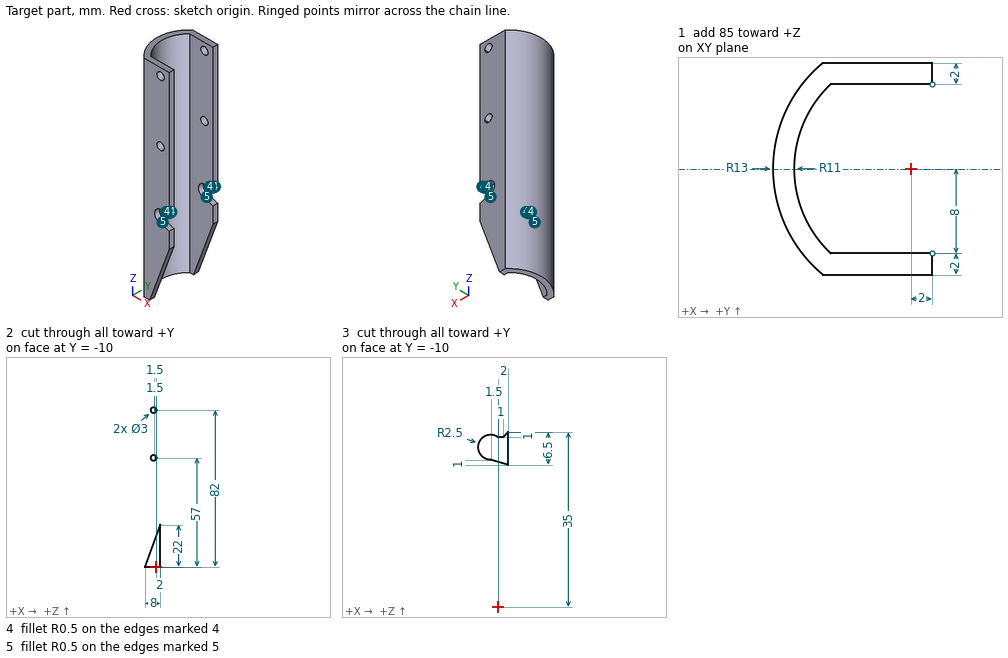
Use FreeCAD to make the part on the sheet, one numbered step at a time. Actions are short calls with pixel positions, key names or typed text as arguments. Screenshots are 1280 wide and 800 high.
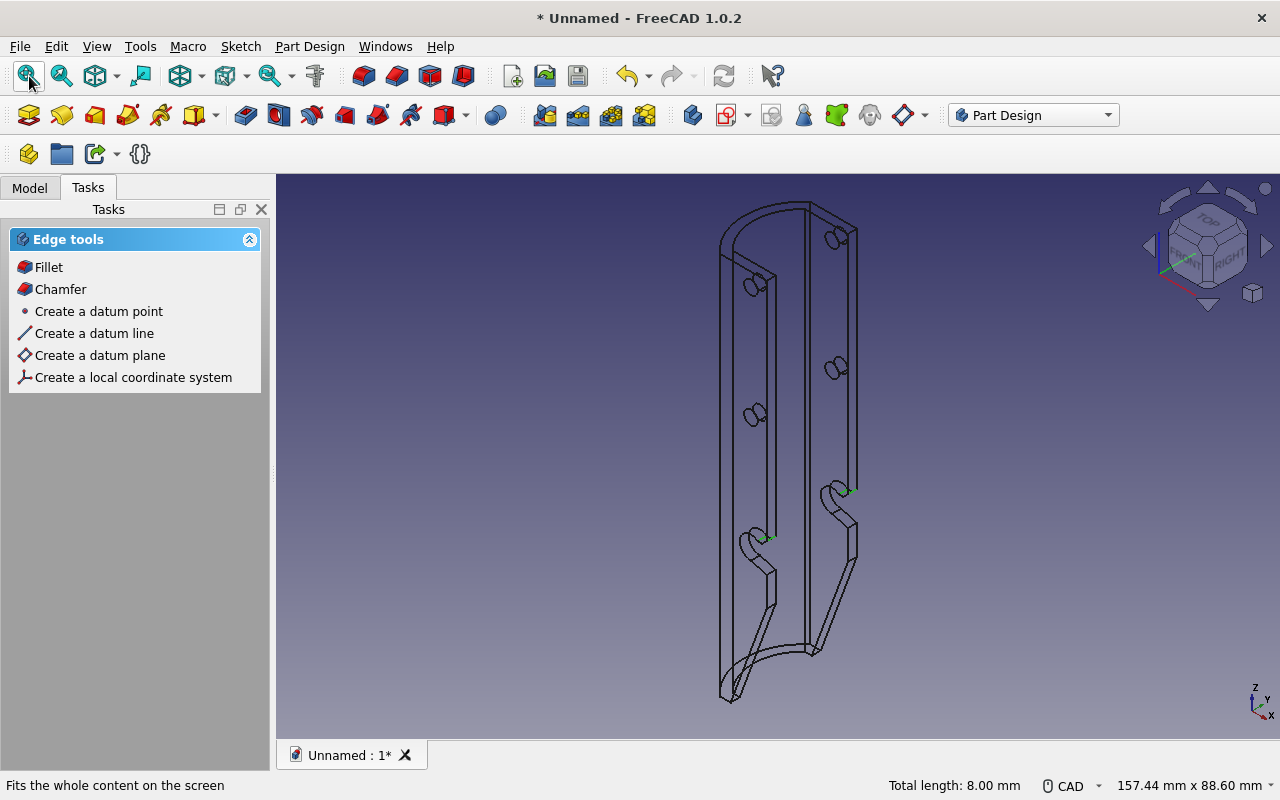
key(2)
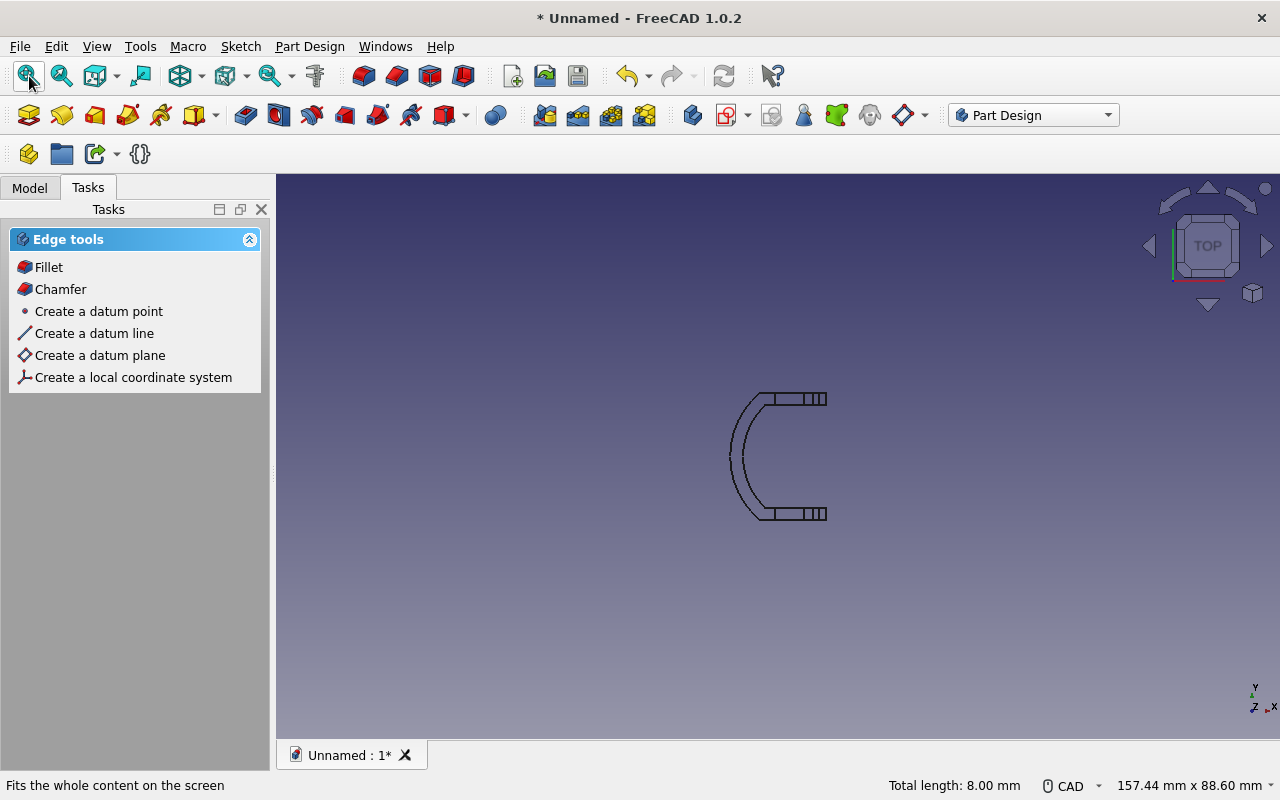
click(29, 76)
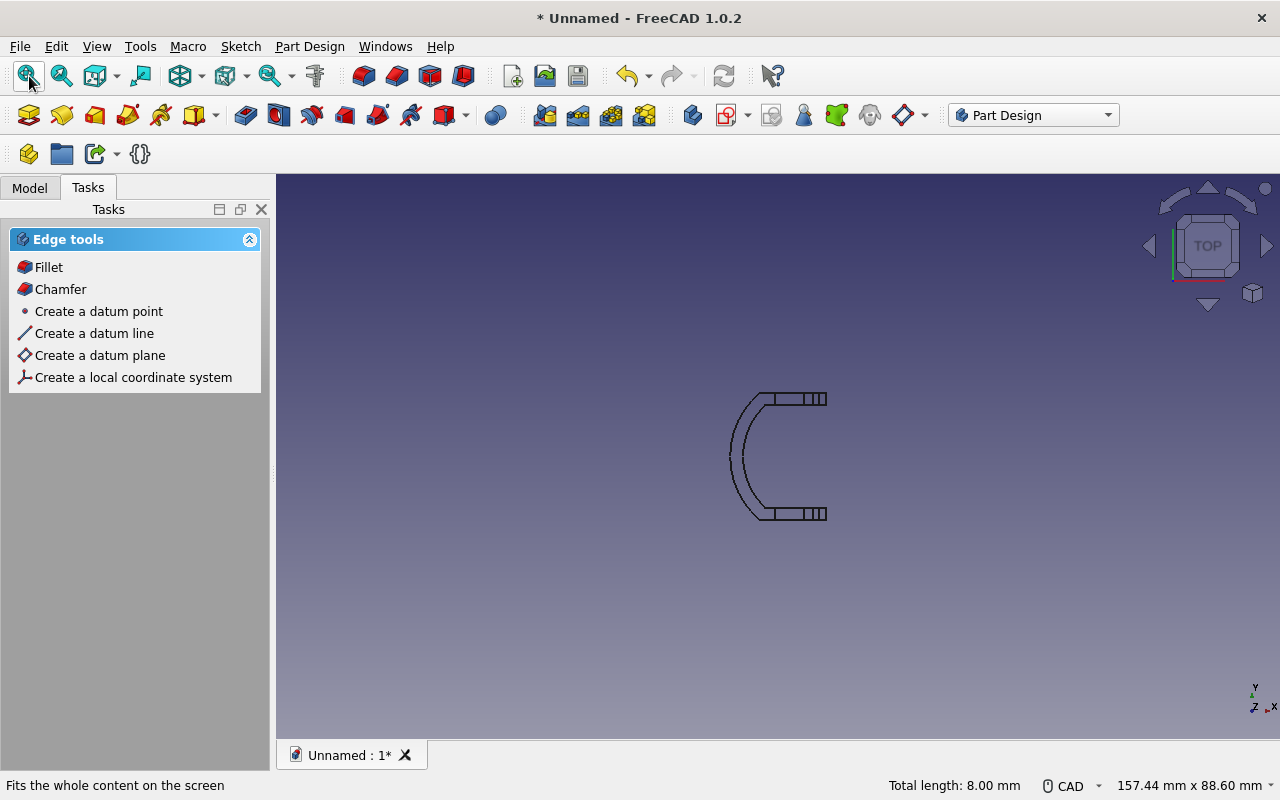
scroll(819, 513, up, 6)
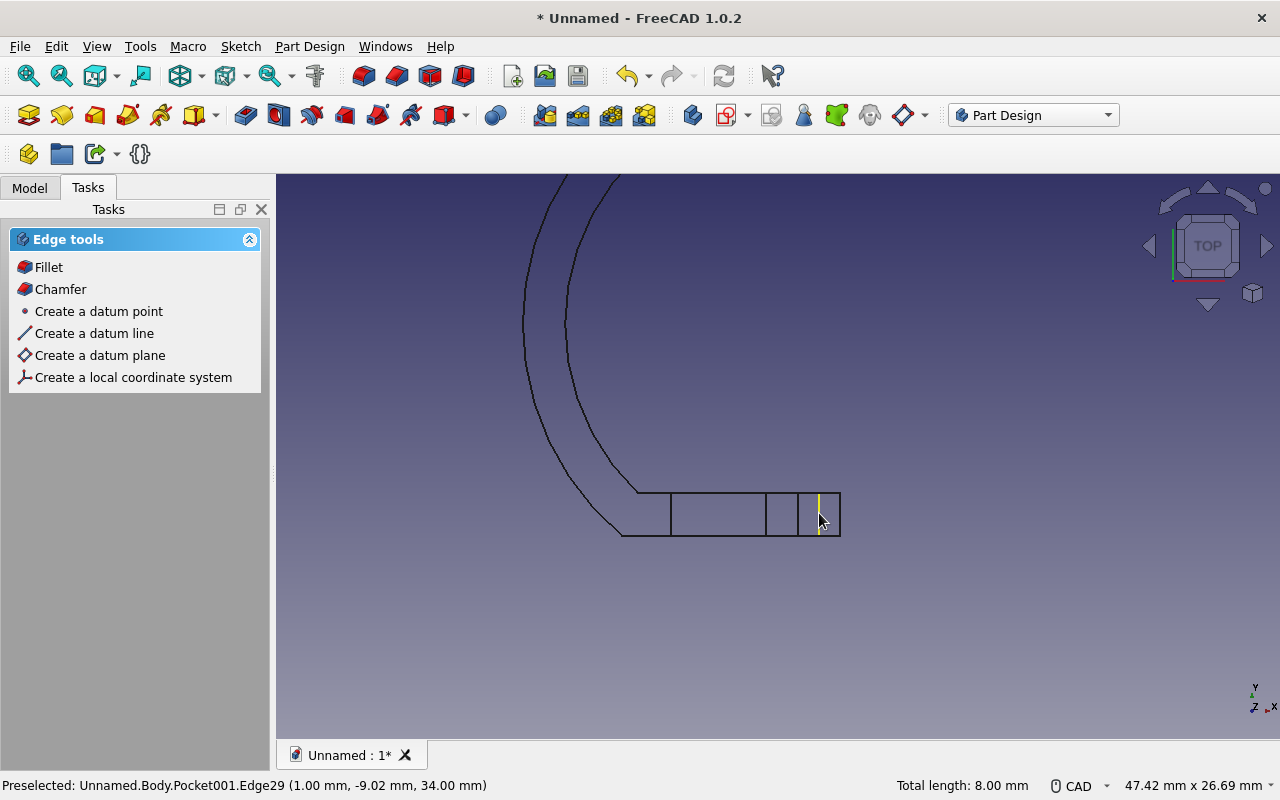
click(819, 514, ctrl)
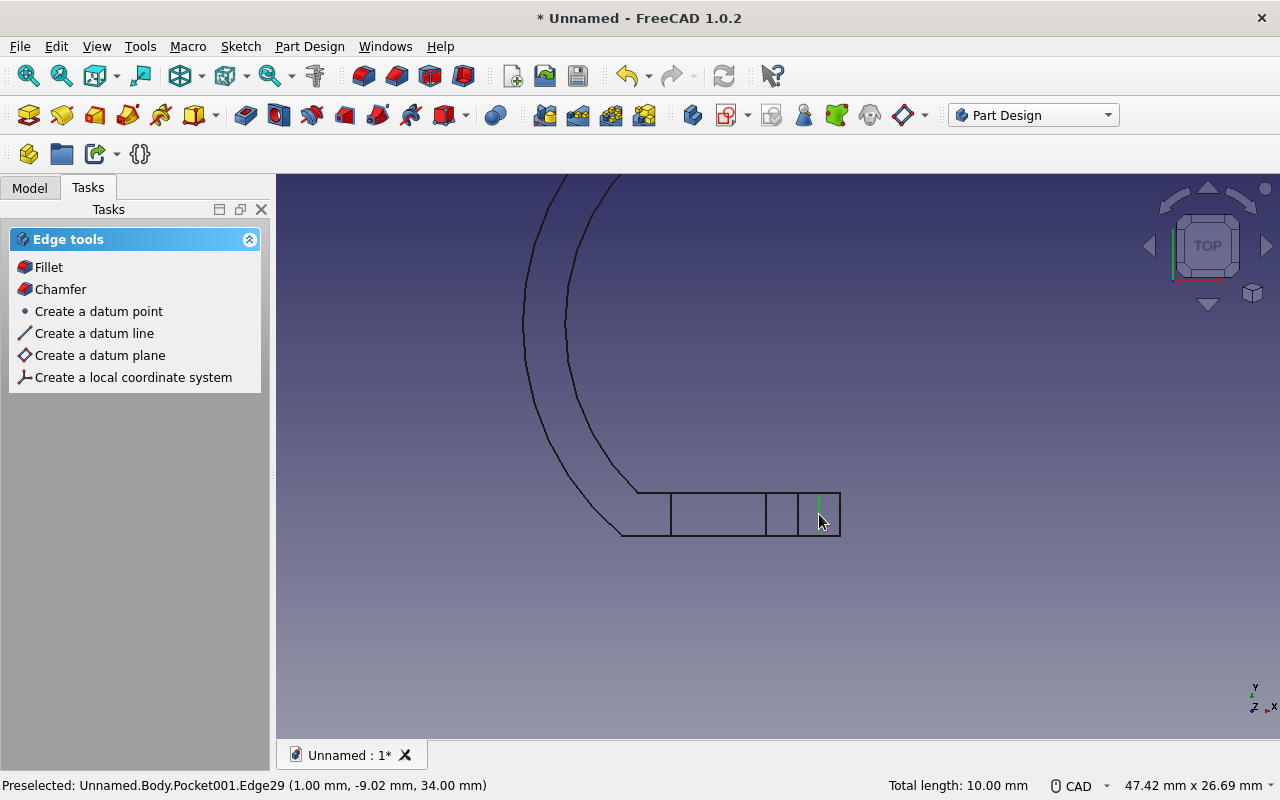
key(v)
key(f)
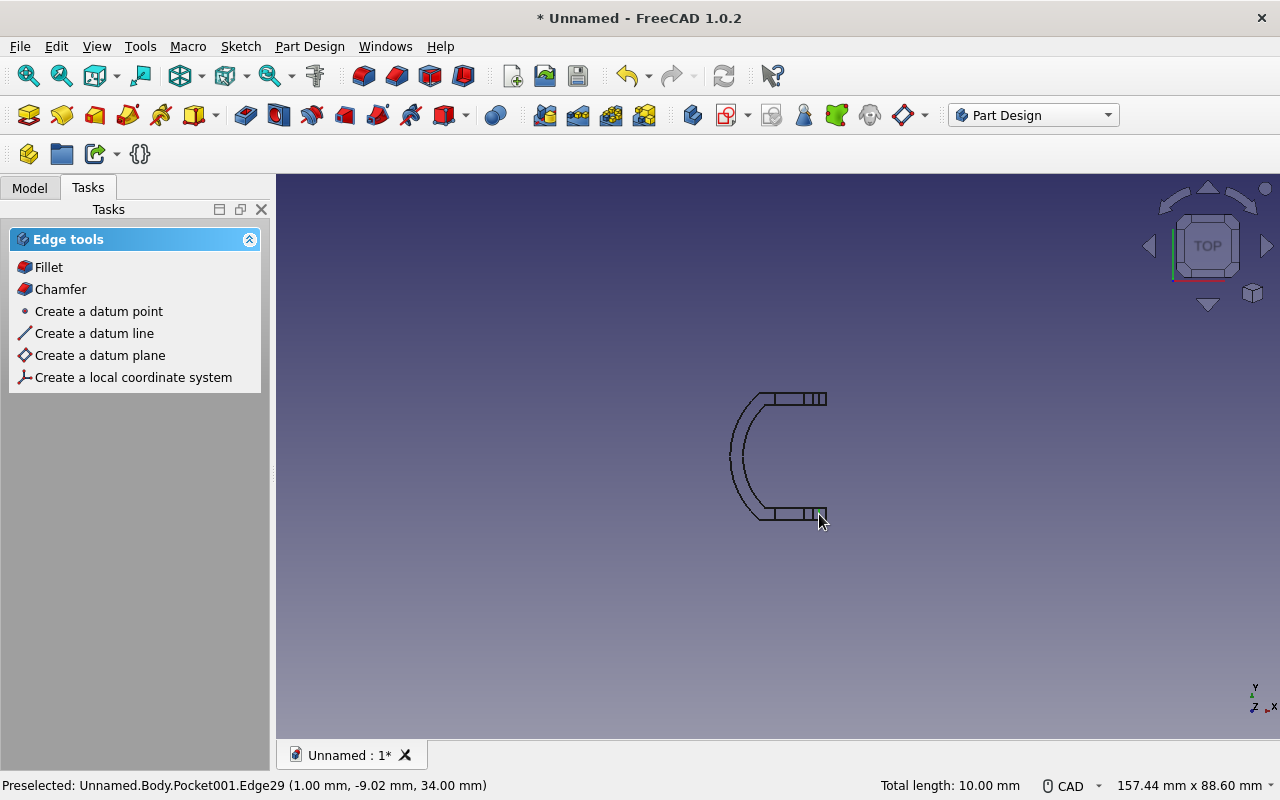
key(1)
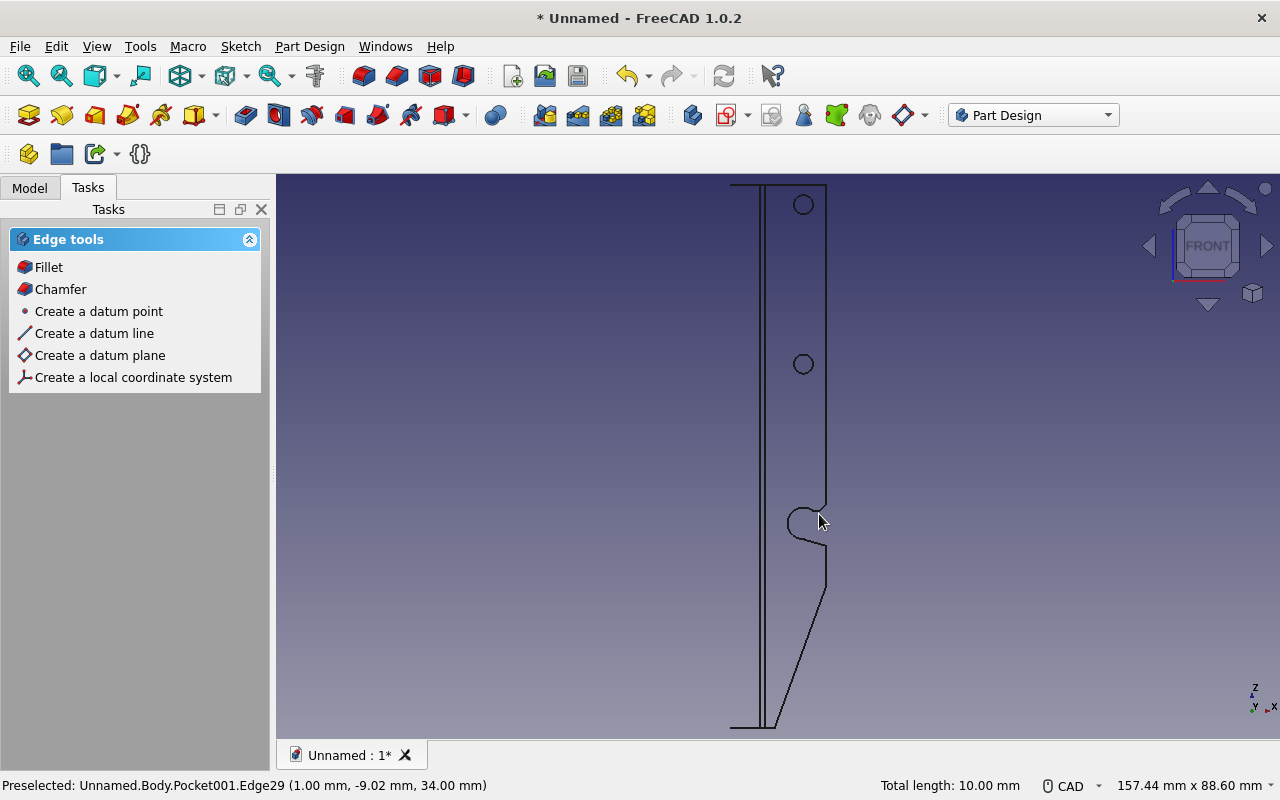
scroll(819, 510, up, 6)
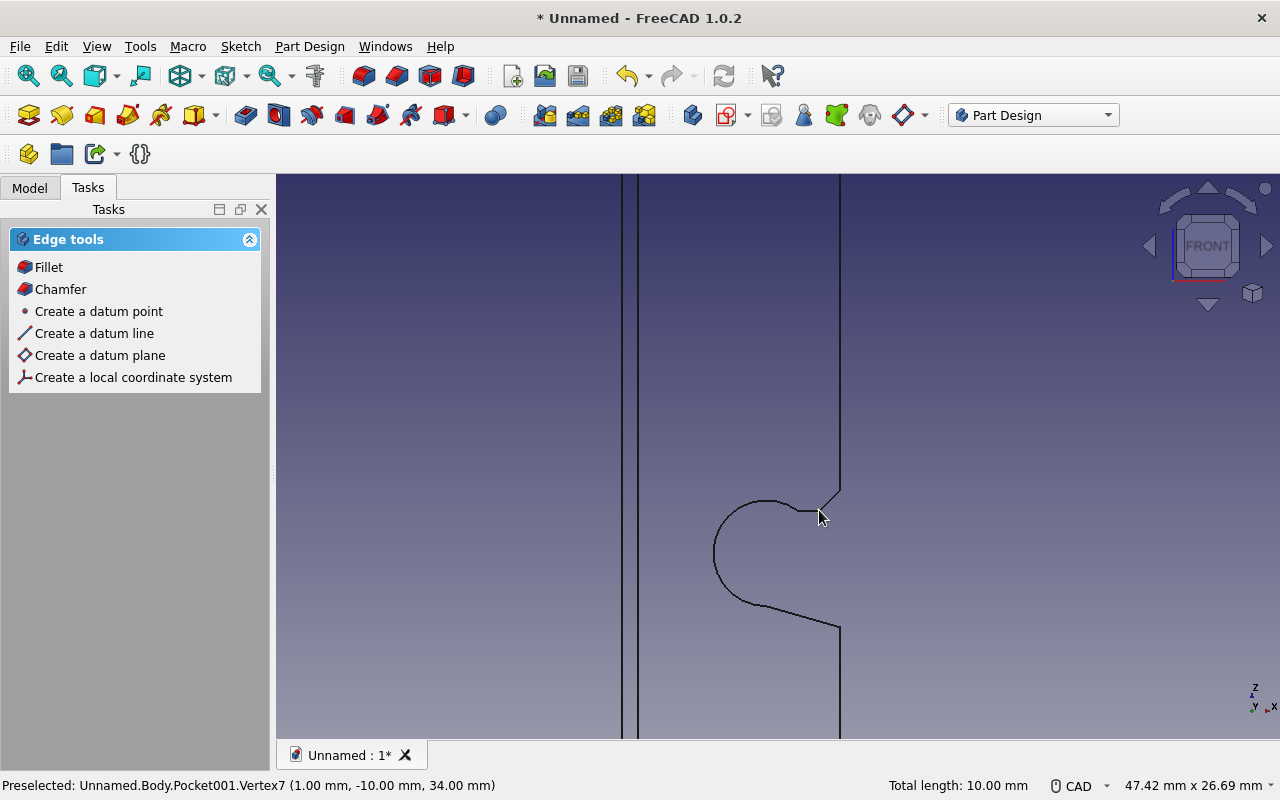
click(29, 76)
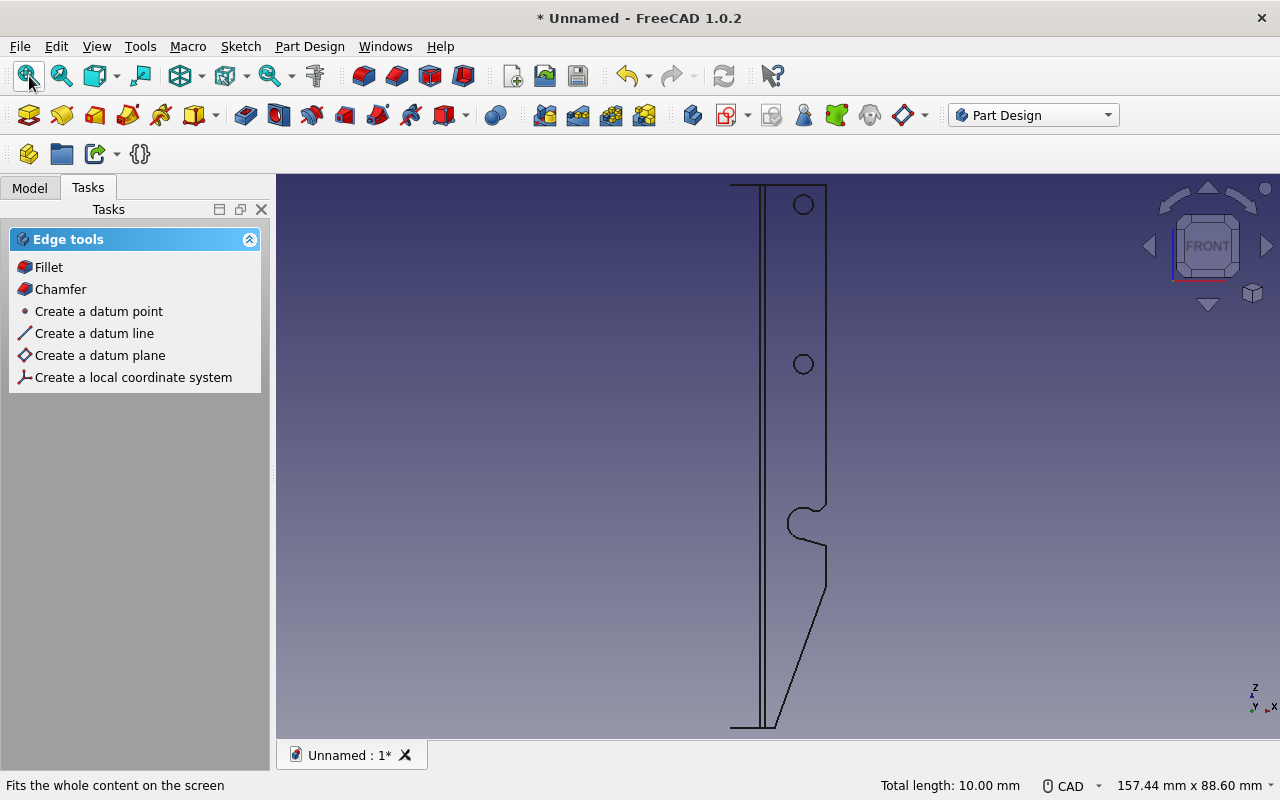
key(3)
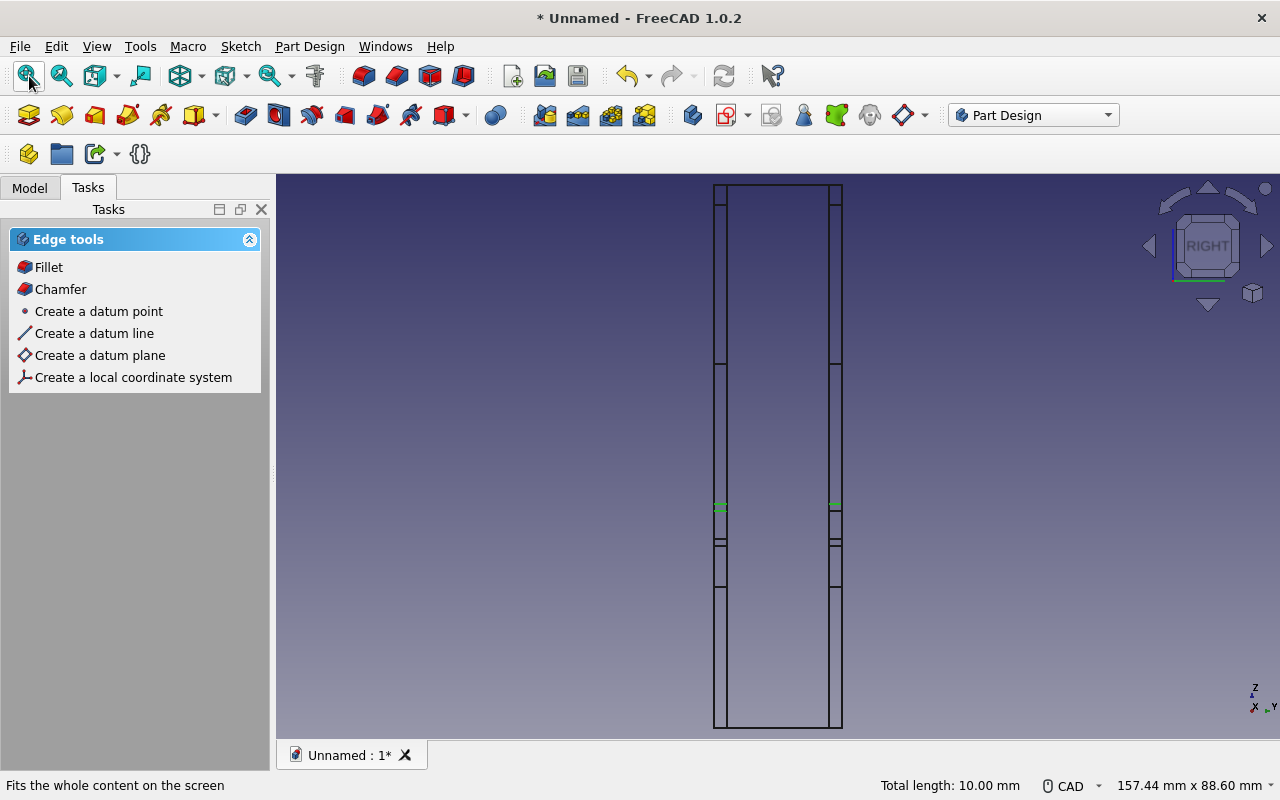
scroll(835, 510, up, 6)